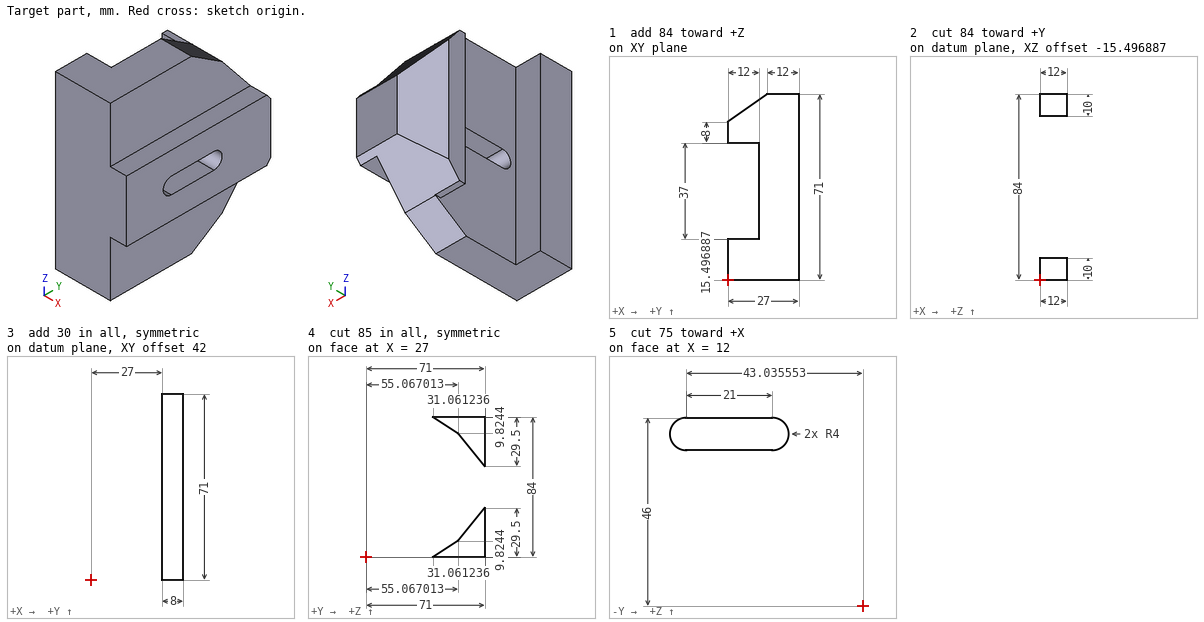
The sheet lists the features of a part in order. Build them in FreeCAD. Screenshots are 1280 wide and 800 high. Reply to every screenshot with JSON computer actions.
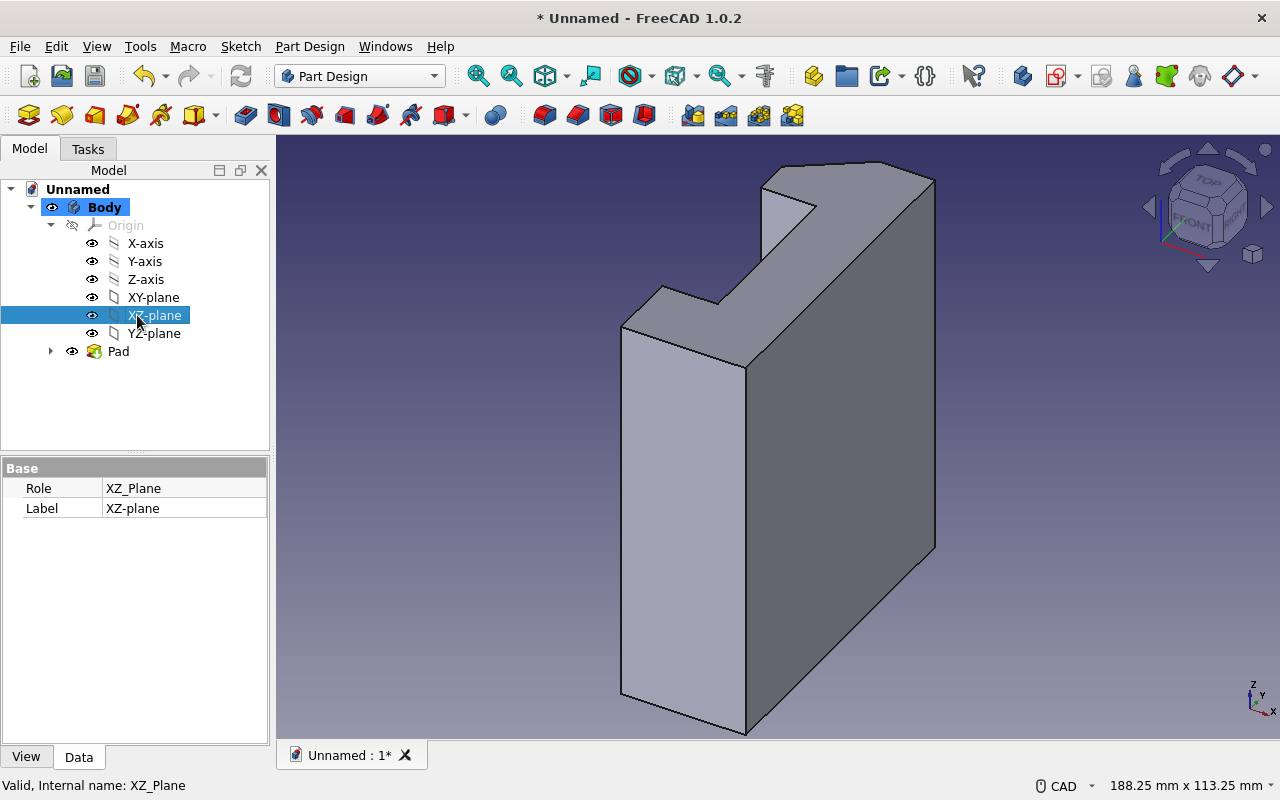
{"action": "left_click", "coordinate": [1232, 76]}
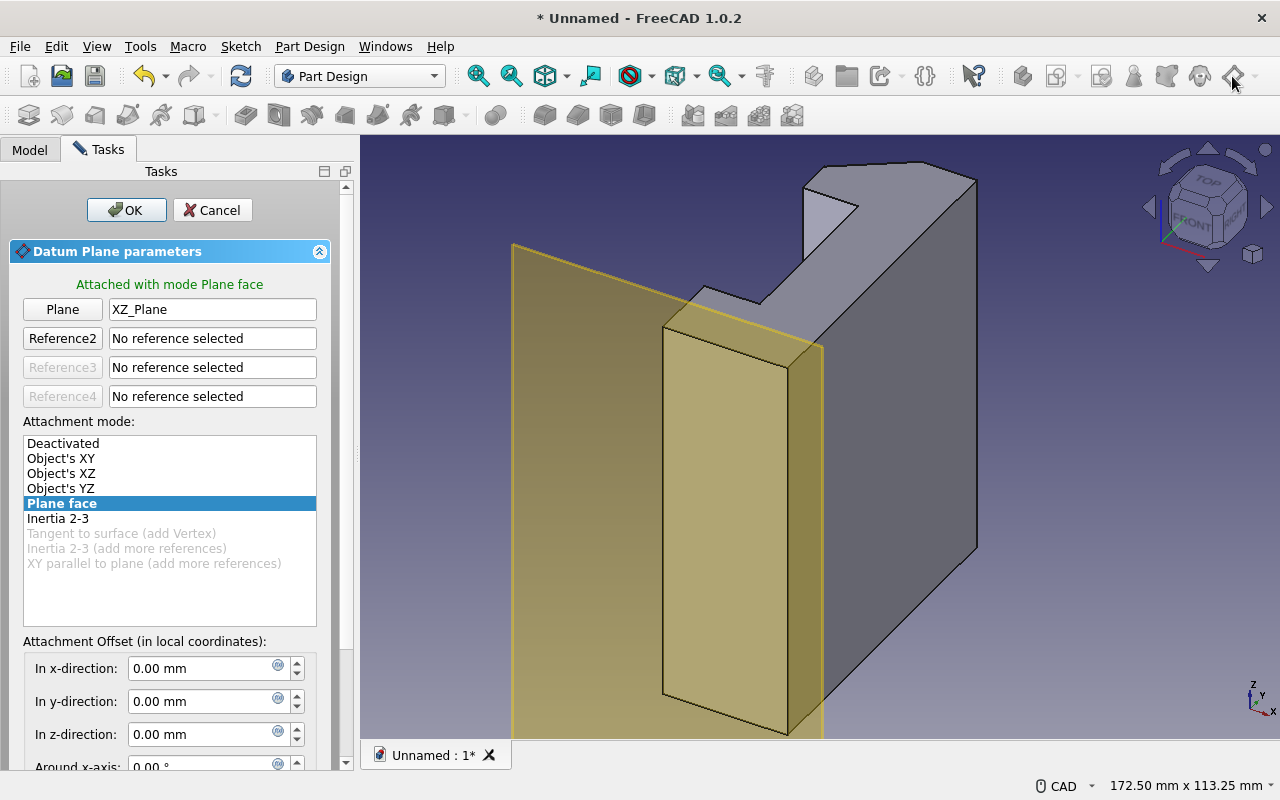
{"action": "triple_click", "coordinate": [210, 734]}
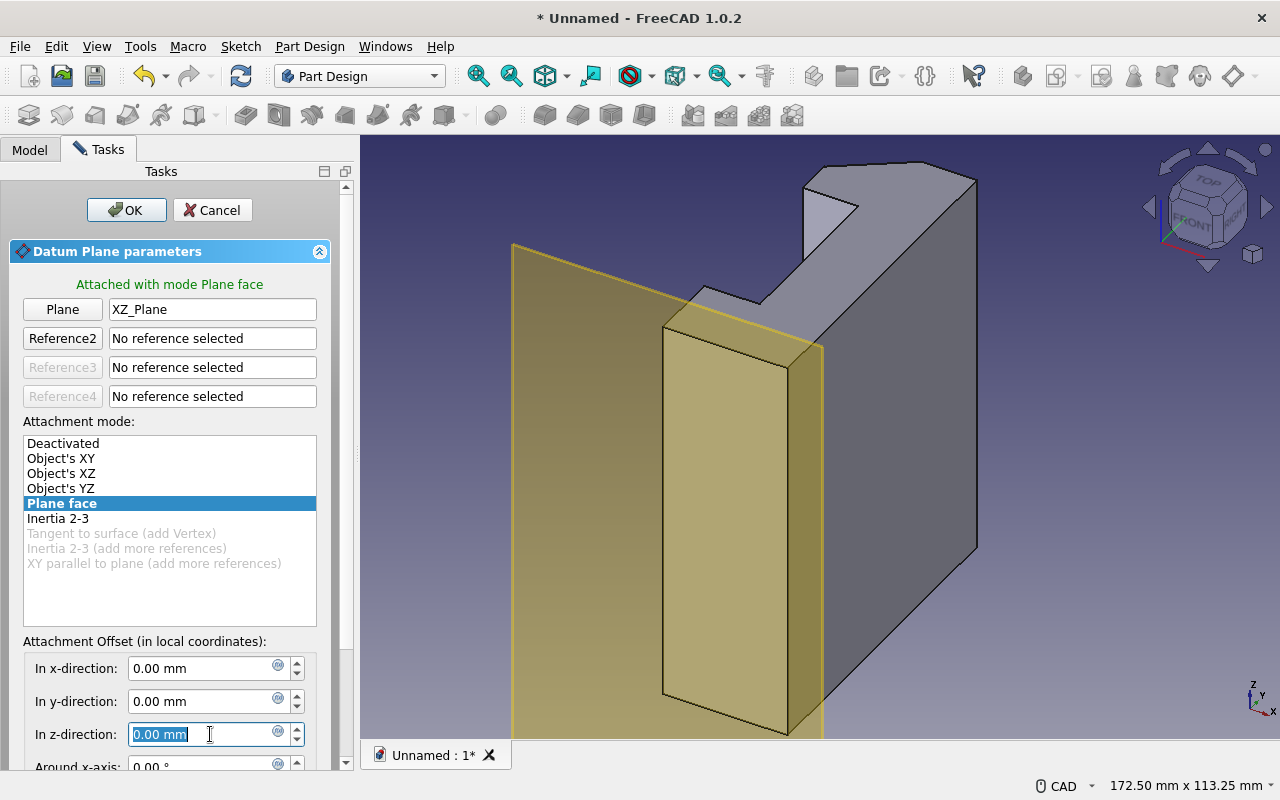
{"action": "type", "text": "-15.496887"}
{"action": "key", "text": "Tab"}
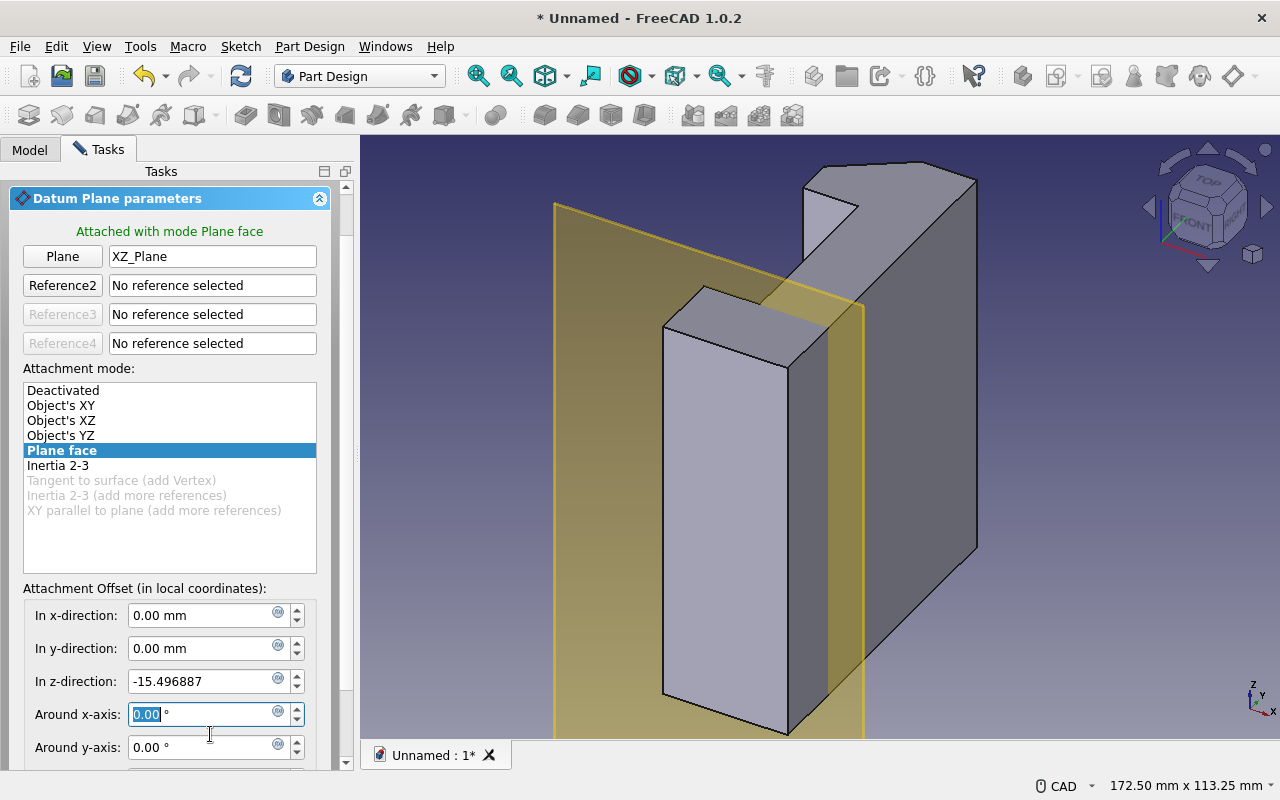
{"action": "scroll", "coordinate": [346, 476], "scroll_direction": "up", "scroll_amount": 2}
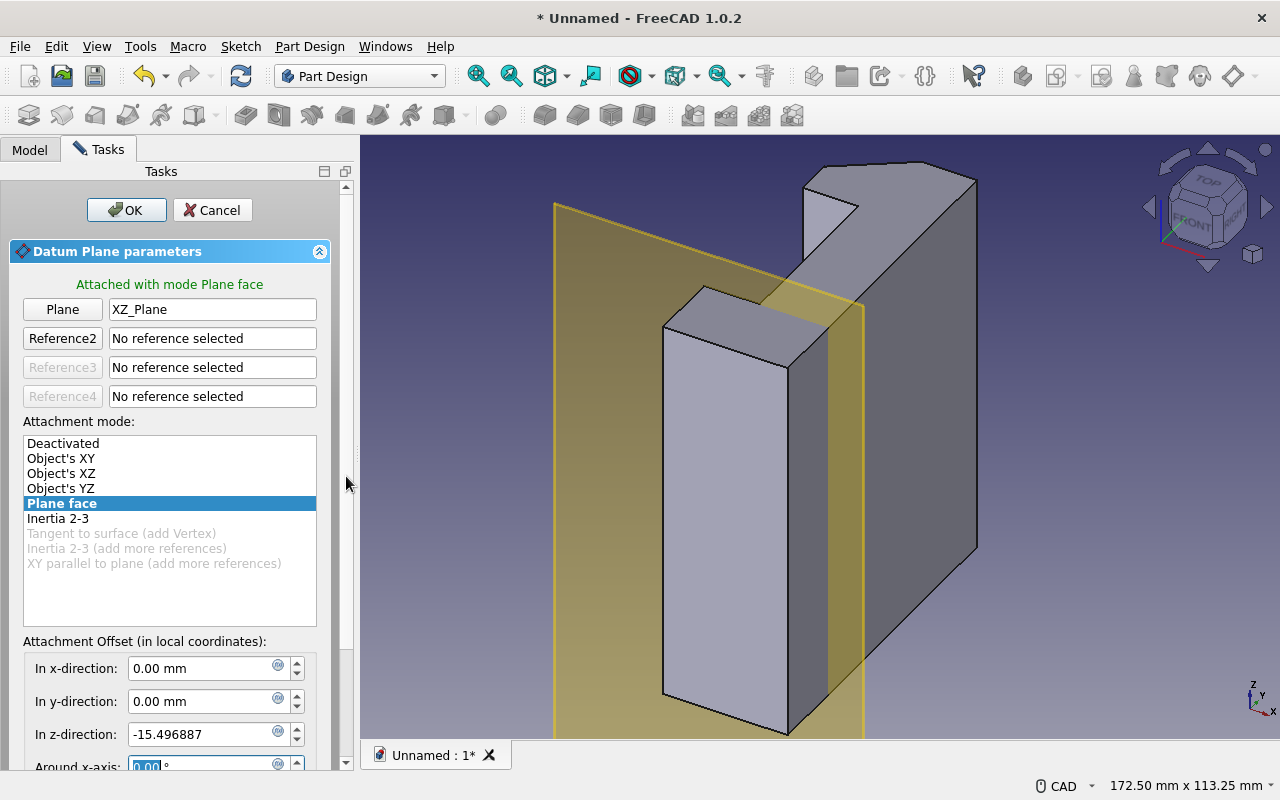
{"action": "left_click", "coordinate": [127, 210]}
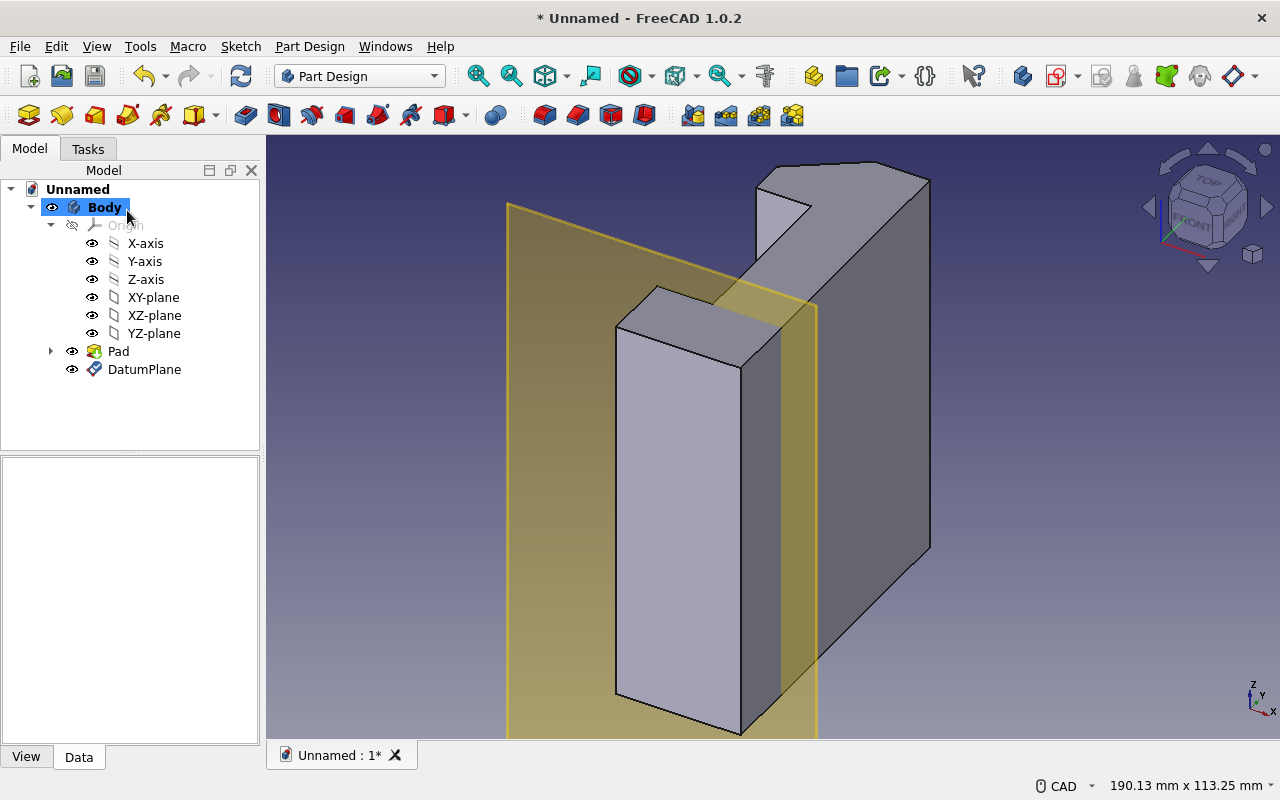
{"action": "left_click", "coordinate": [117, 369]}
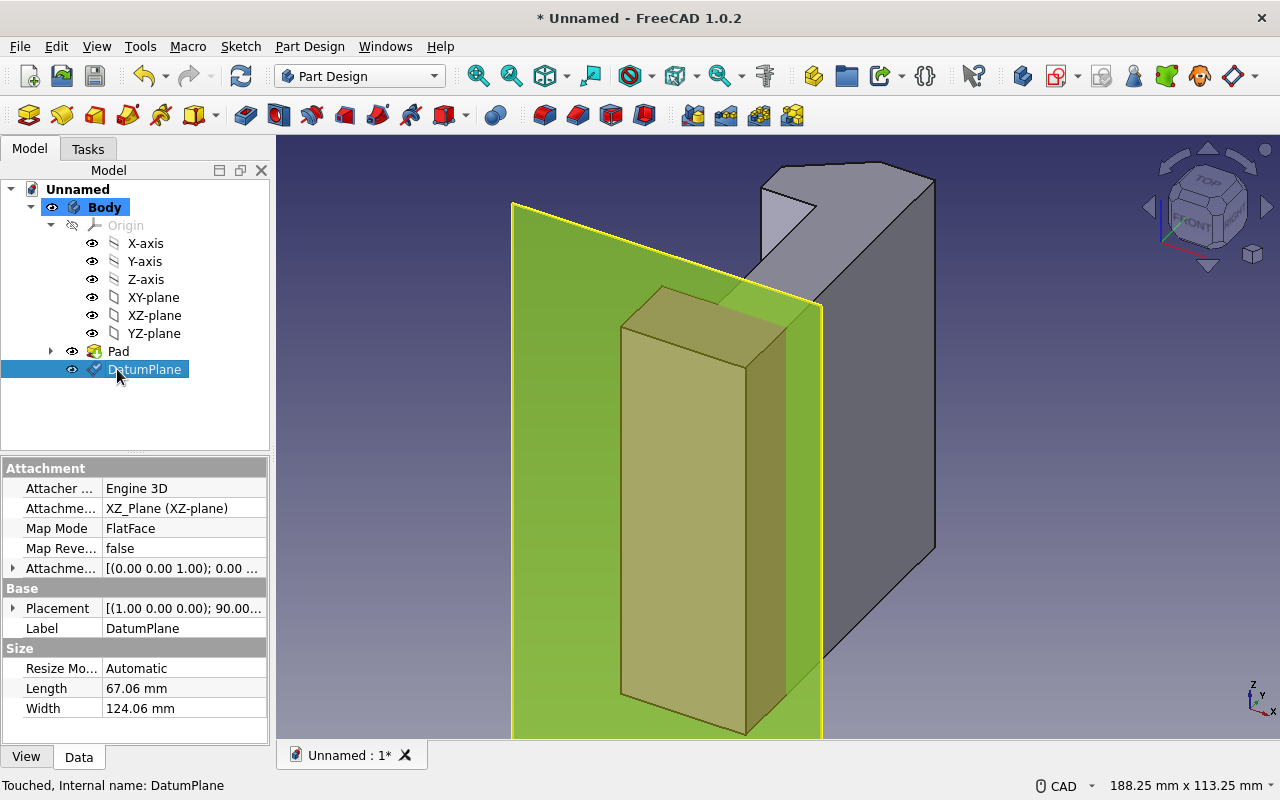
{"action": "left_click", "coordinate": [1056, 76]}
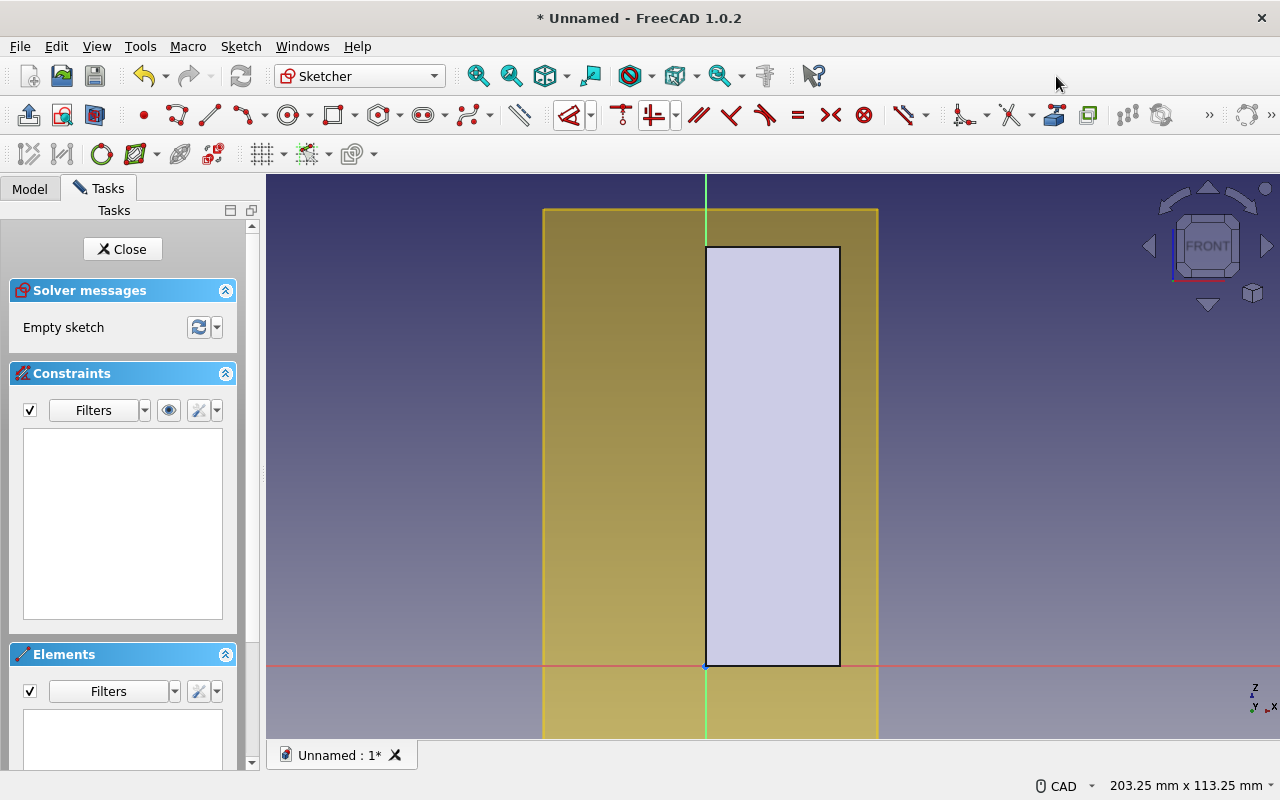
{"action": "left_click", "coordinate": [95, 116]}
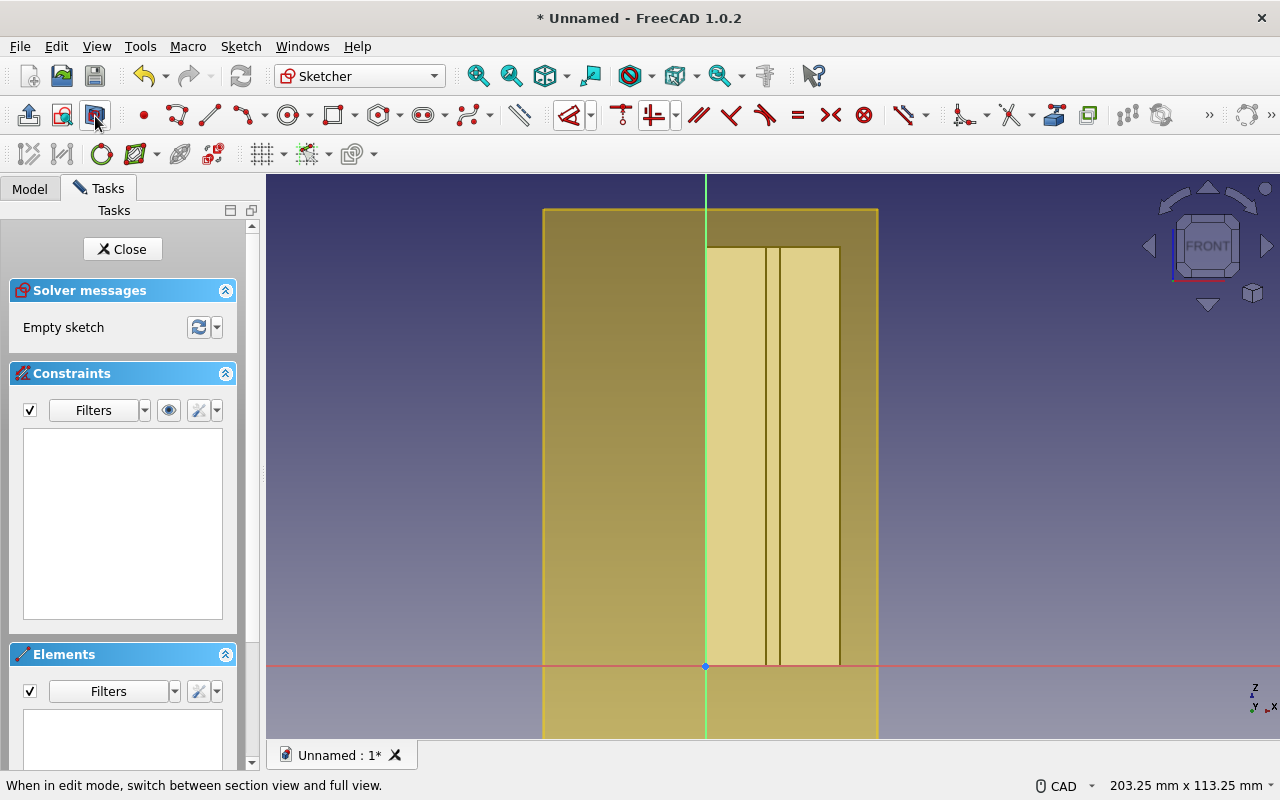
{"action": "left_click", "coordinate": [332, 116]}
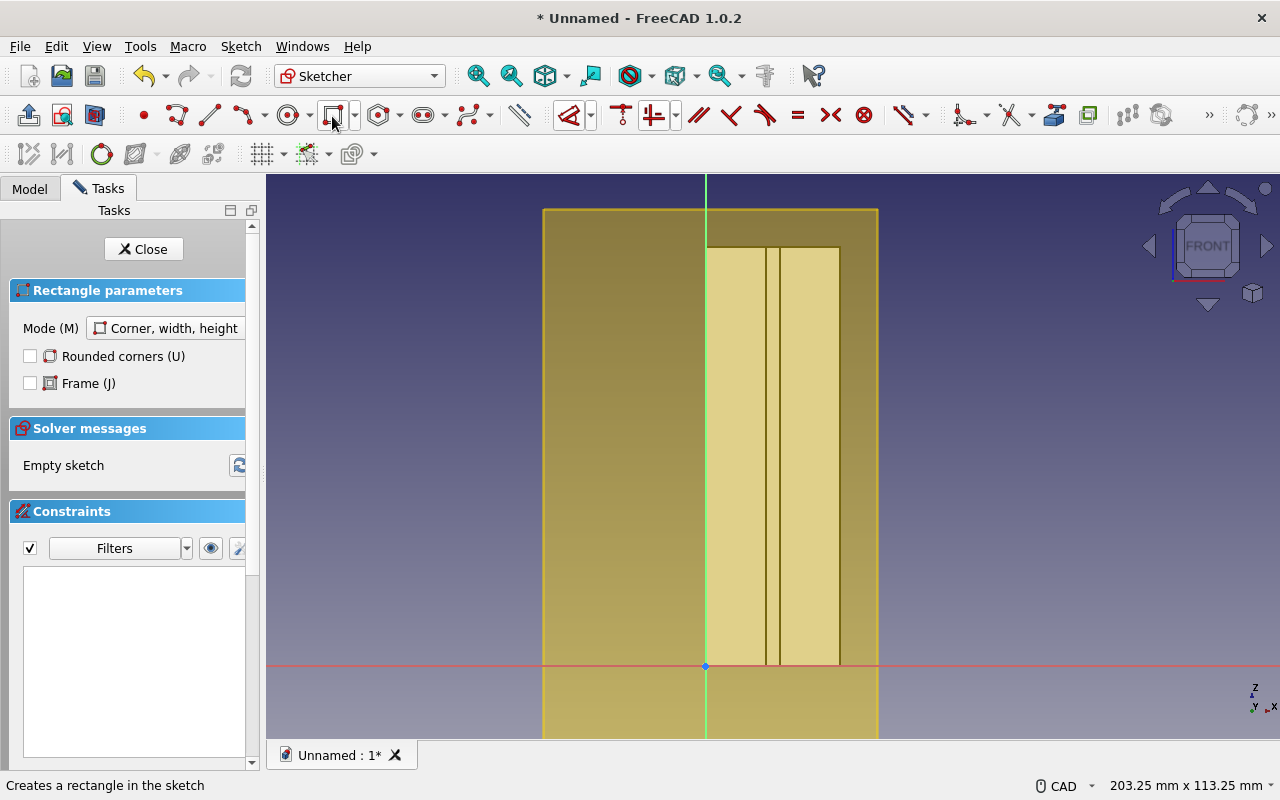
{"action": "left_click", "coordinate": [706, 247]}
{"action": "mouse_move", "coordinate": [766, 297]}